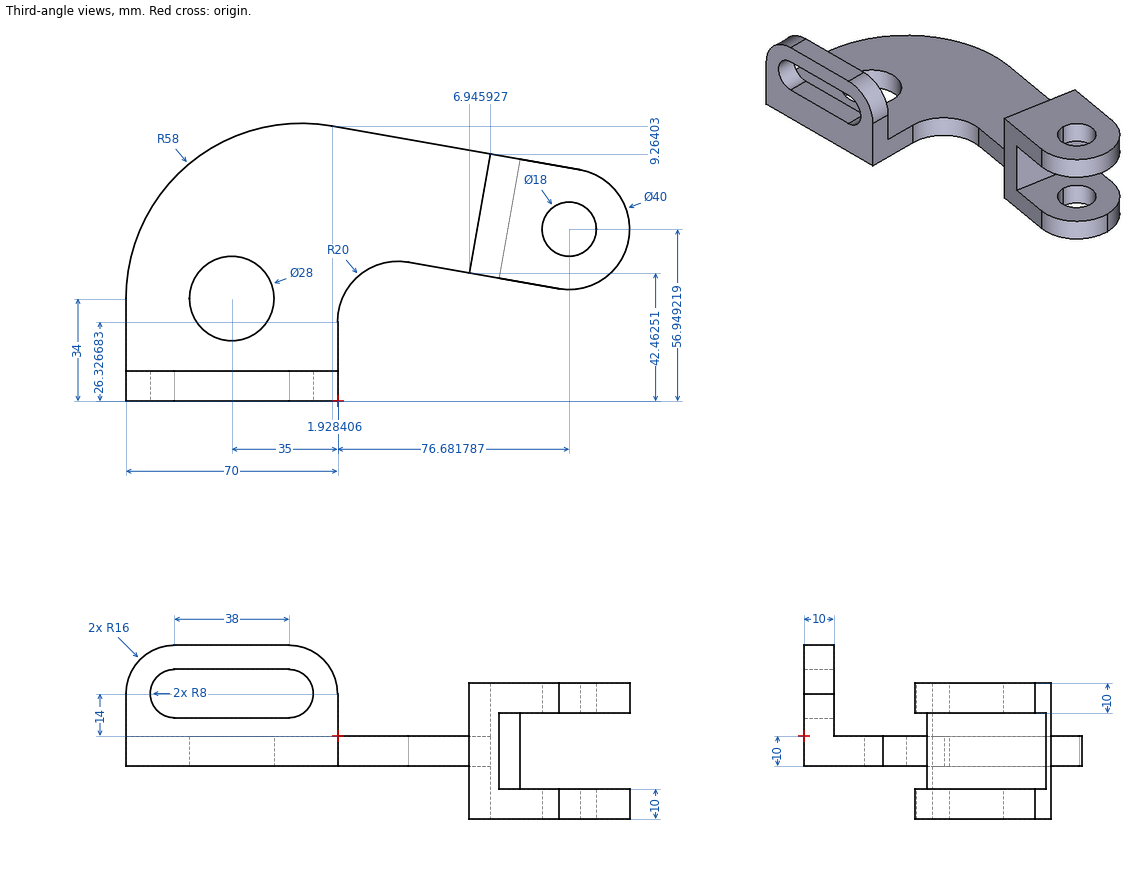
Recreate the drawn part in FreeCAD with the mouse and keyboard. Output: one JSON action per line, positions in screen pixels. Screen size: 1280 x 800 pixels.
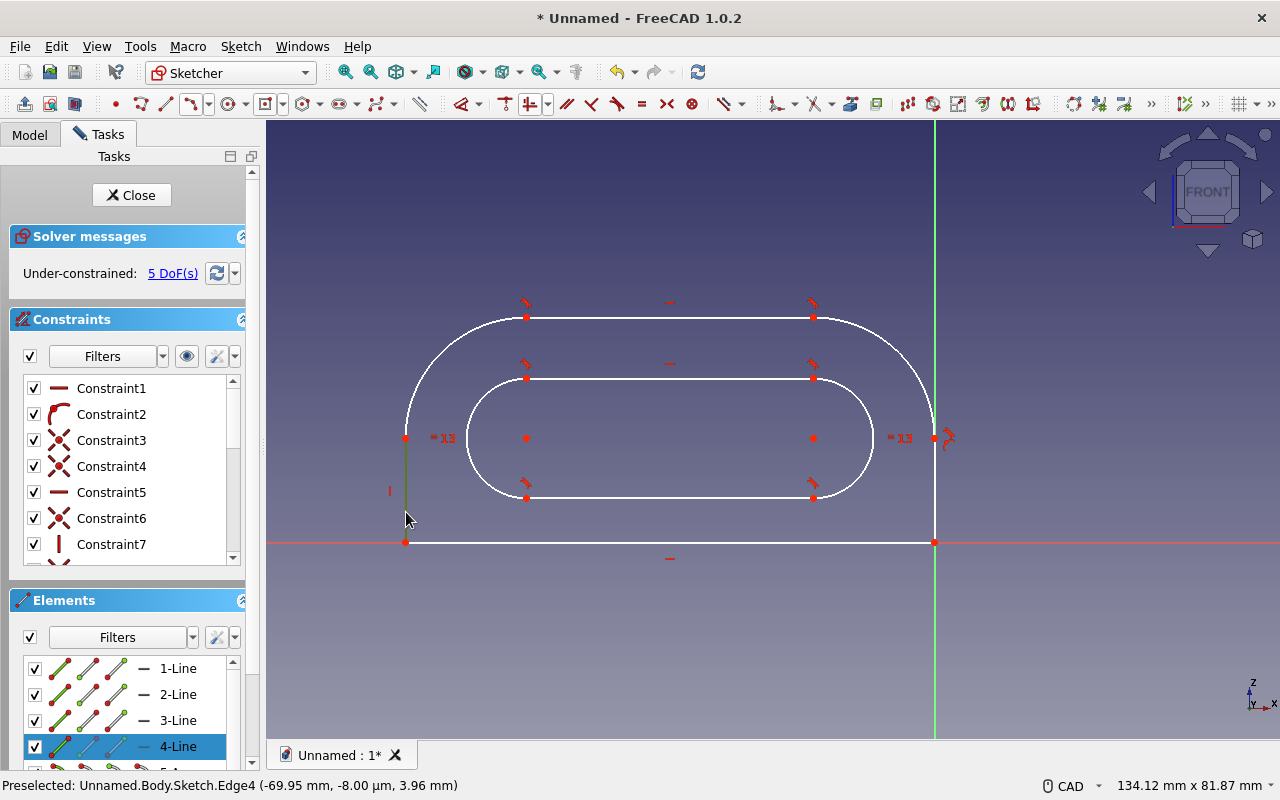
{"action": "left_click", "coordinate": [472, 331]}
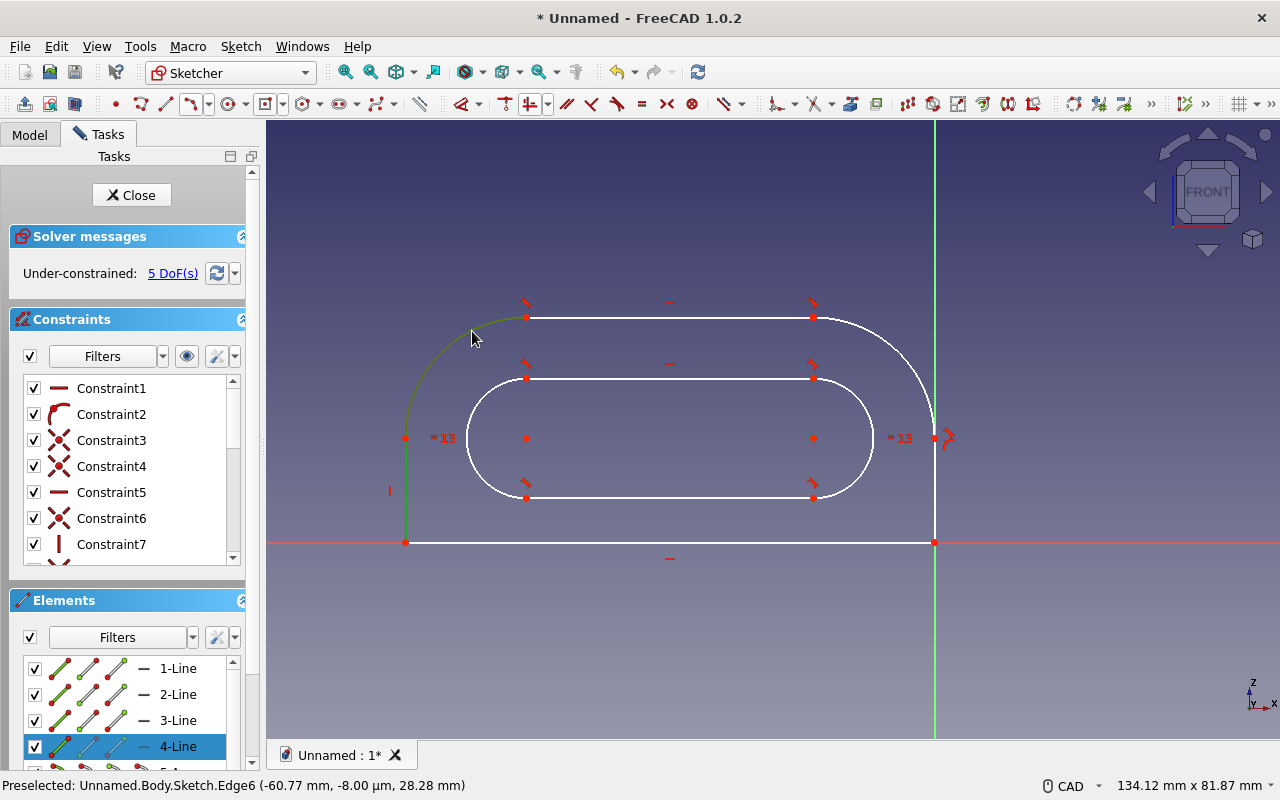
{"action": "left_click", "coordinate": [617, 104]}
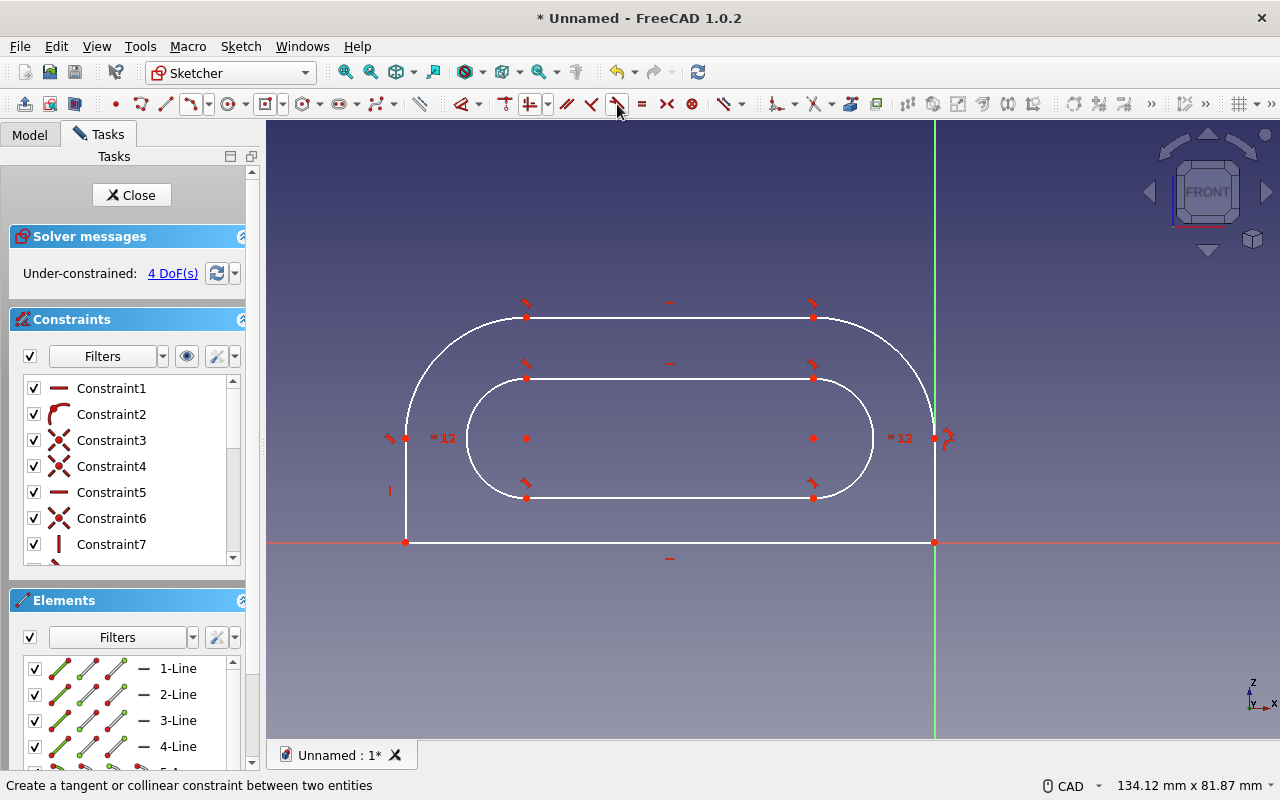
{"action": "left_click", "coordinate": [460, 104]}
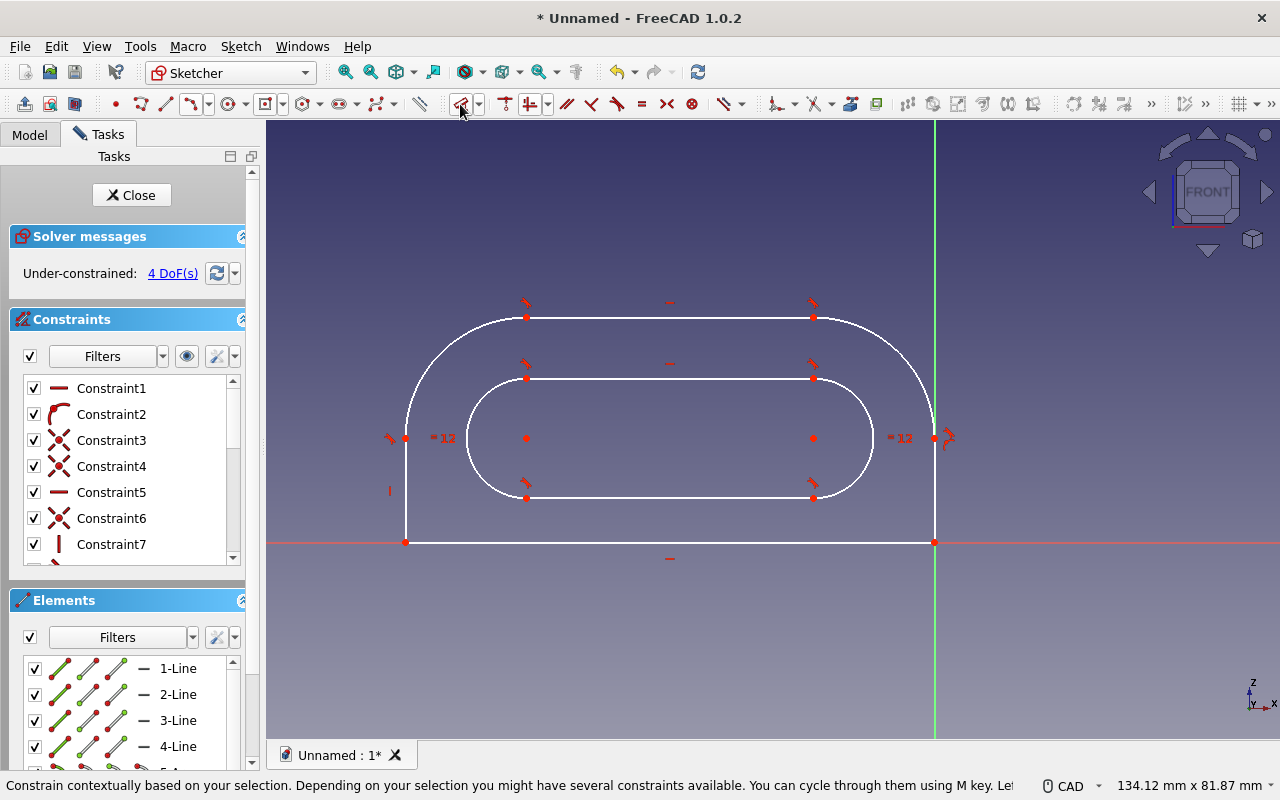
{"action": "left_click", "coordinate": [921, 384]}
{"action": "left_click", "coordinate": [950, 370]}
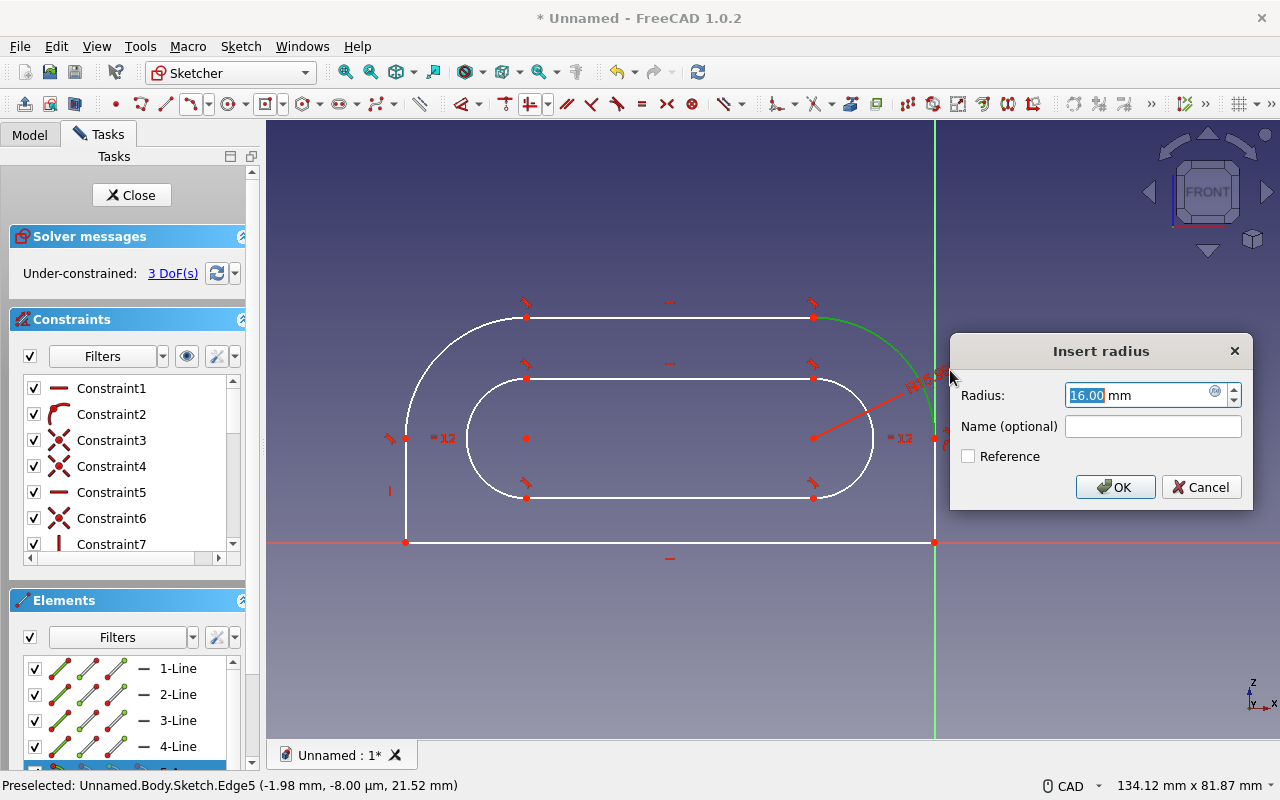
{"action": "type", "text": "16"}
{"action": "key", "text": "Return"}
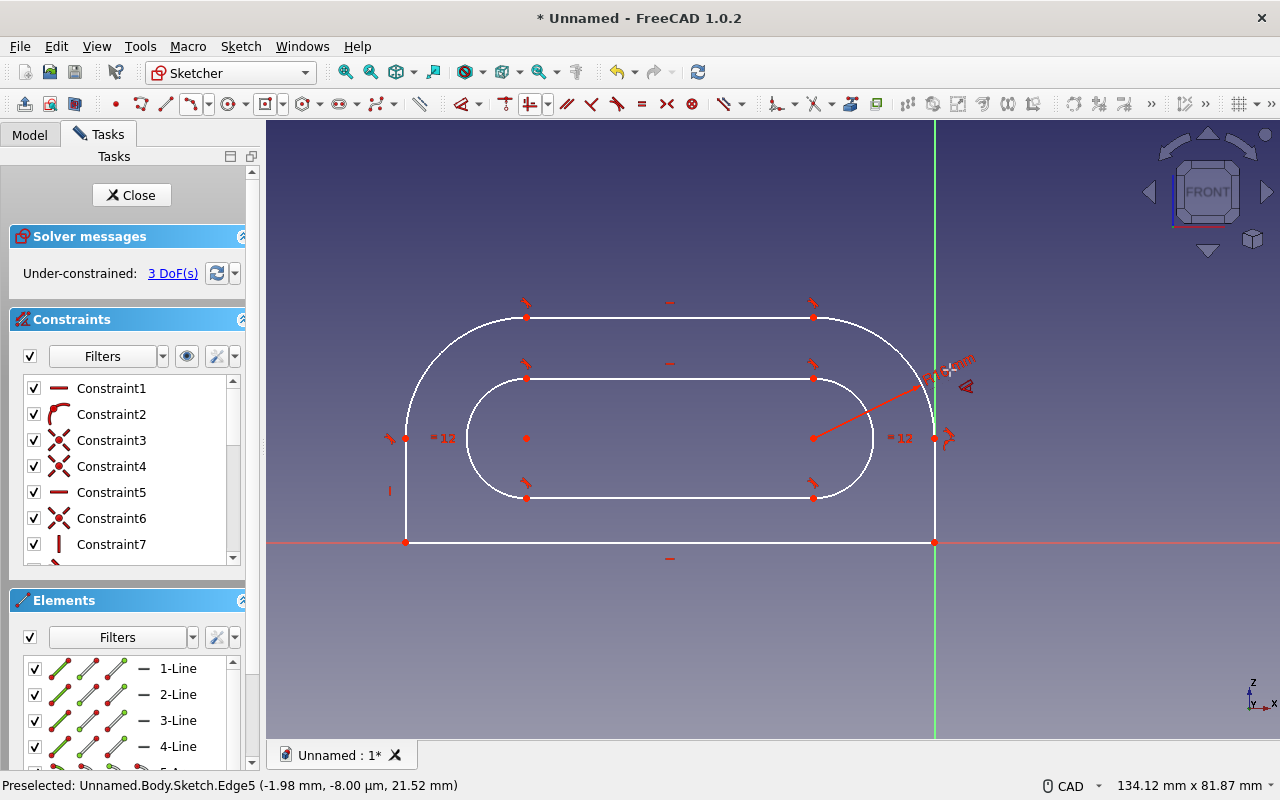
{"action": "left_click", "coordinate": [478, 403]}
{"action": "left_click", "coordinate": [452, 384]}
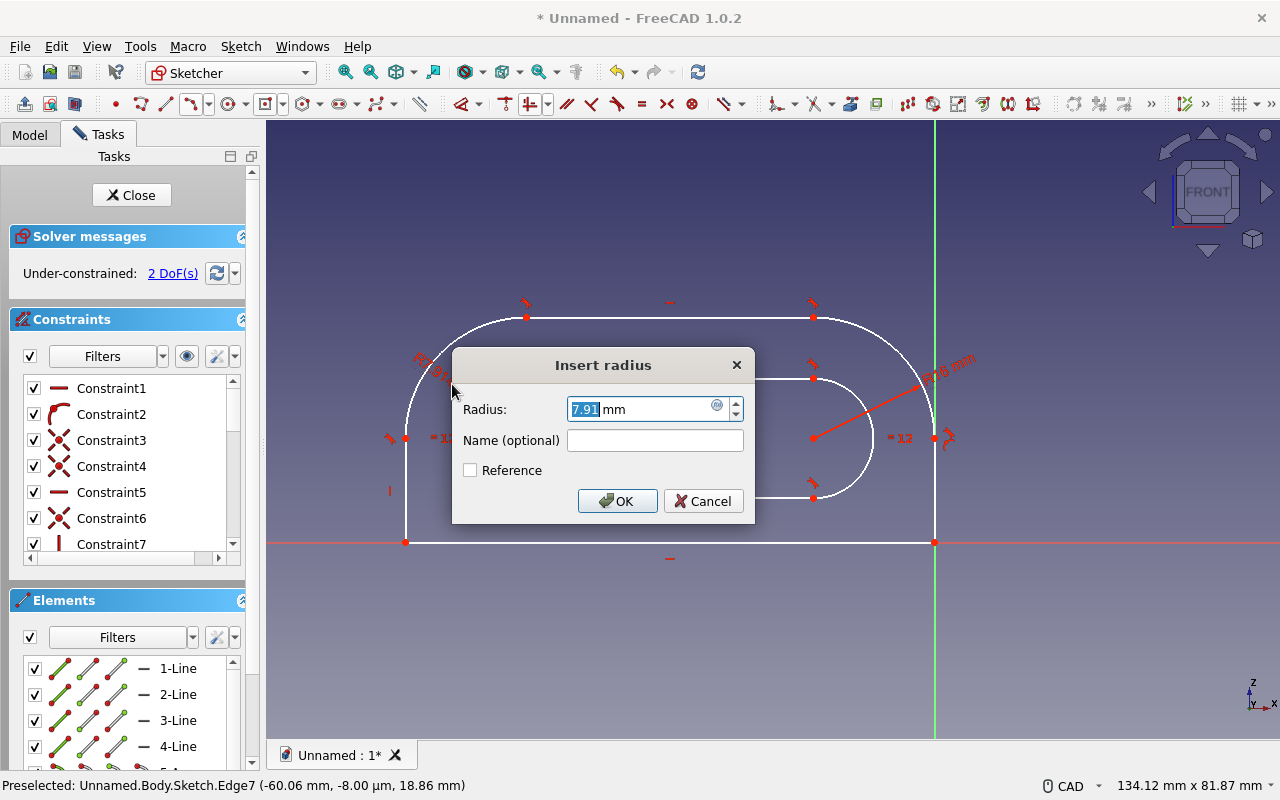
{"action": "type", "text": "8"}
{"action": "key", "text": "Return"}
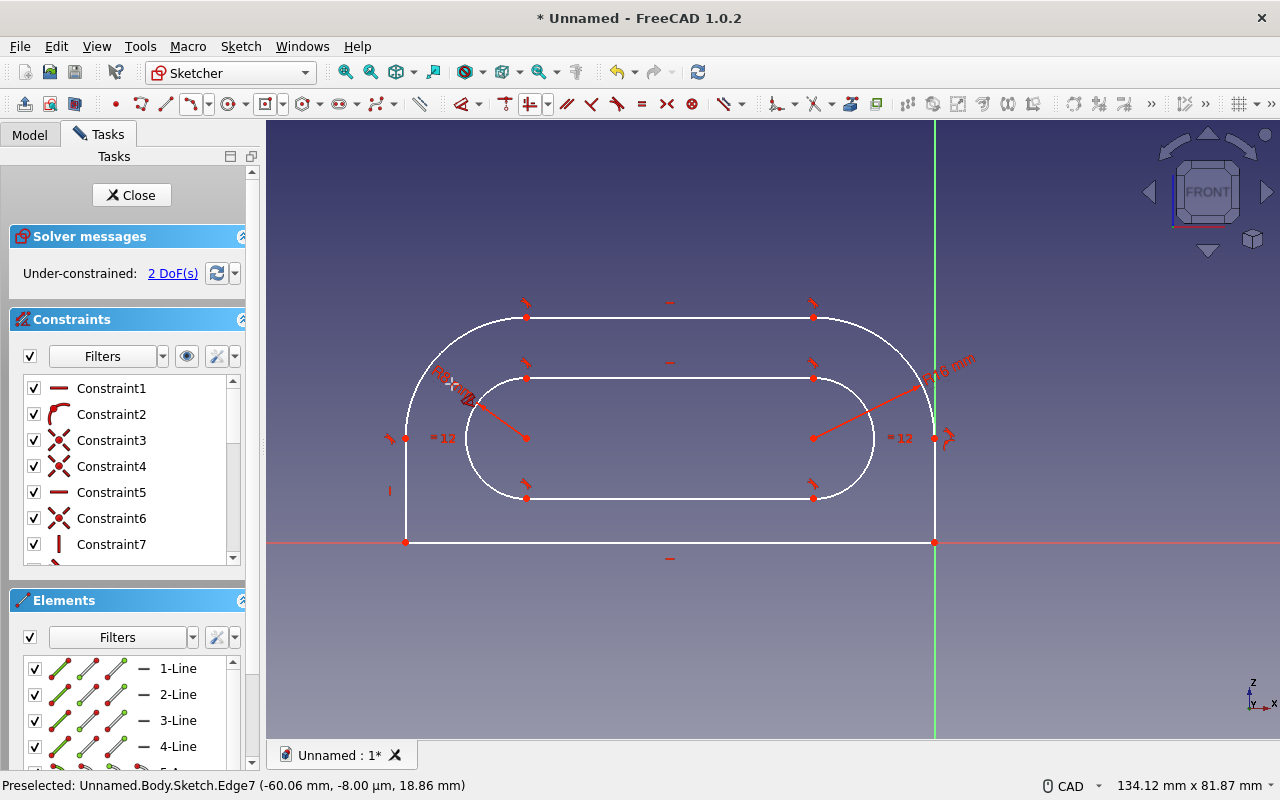
{"action": "left_click", "coordinate": [613, 318]}
{"action": "left_click", "coordinate": [670, 284]}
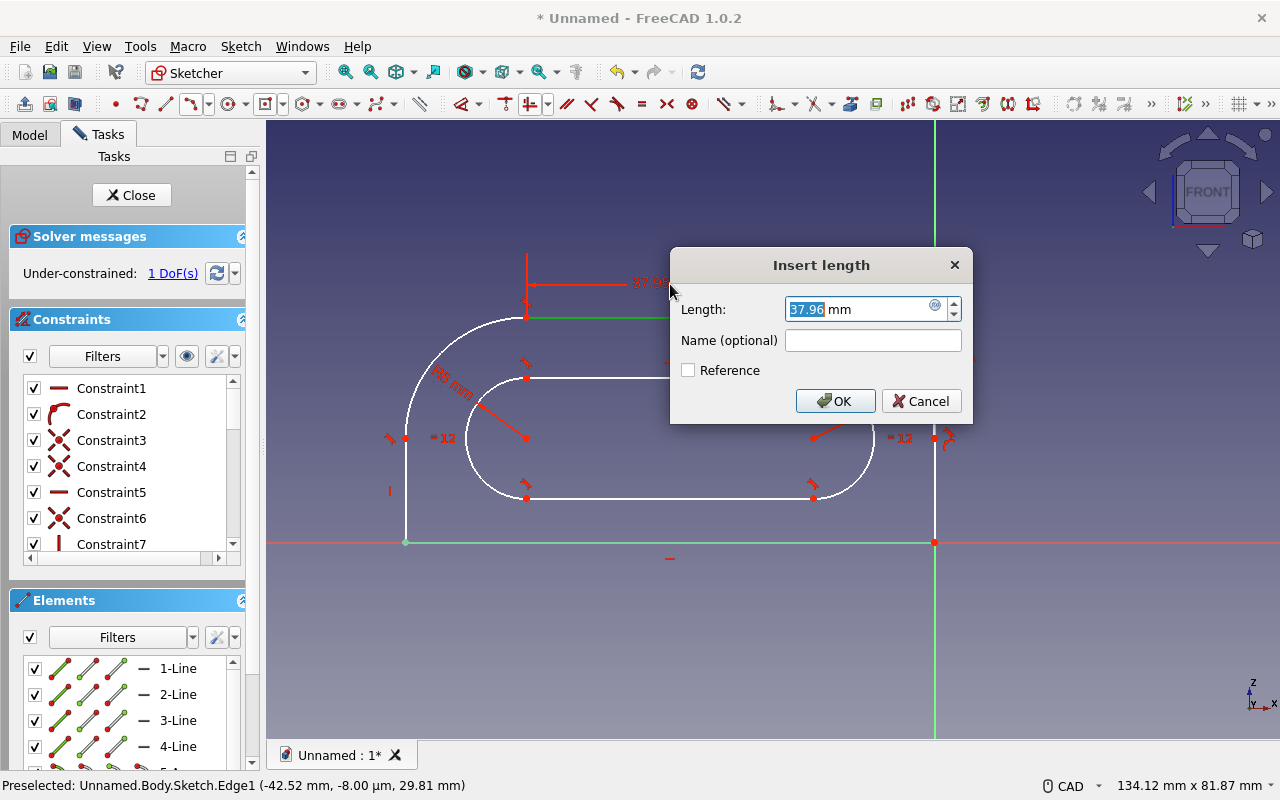
{"action": "type", "text": "38"}
{"action": "key", "text": "Return"}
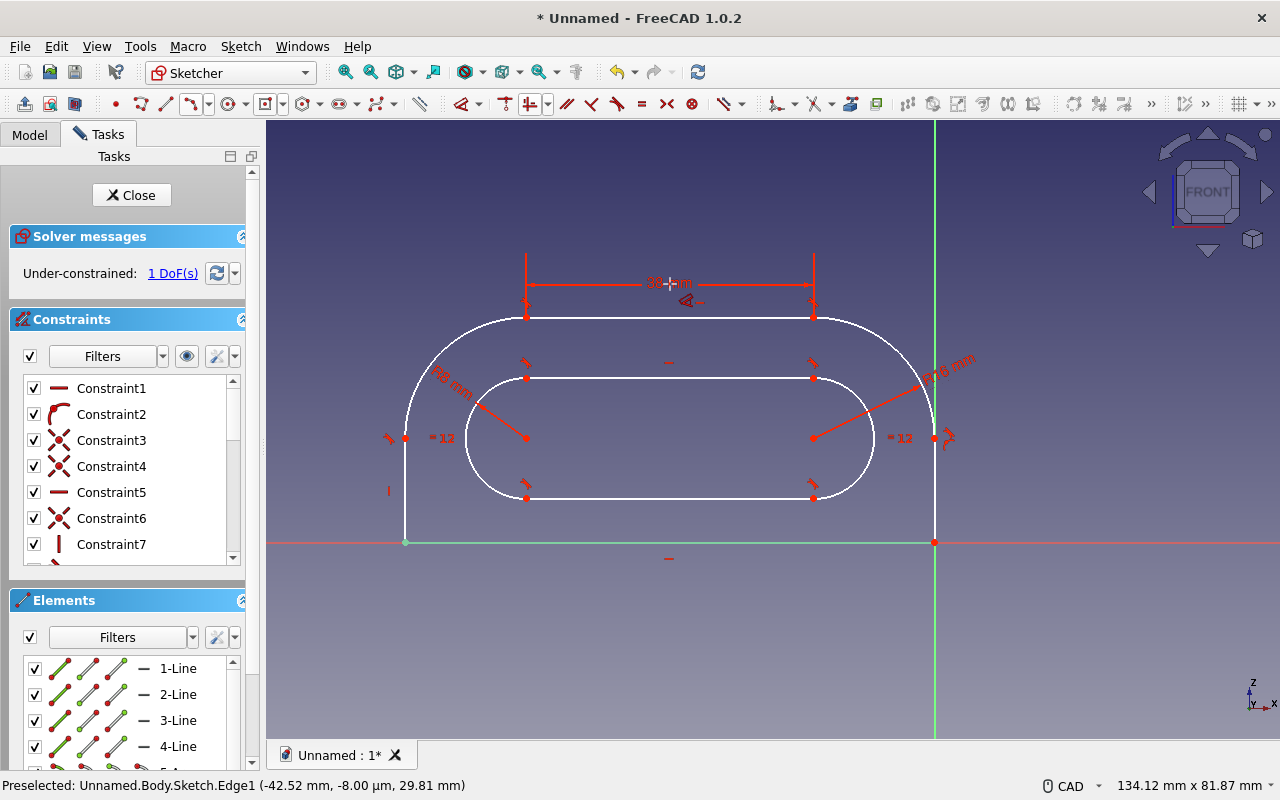
{"action": "left_click", "coordinate": [935, 470]}
{"action": "left_click", "coordinate": [969, 491]}